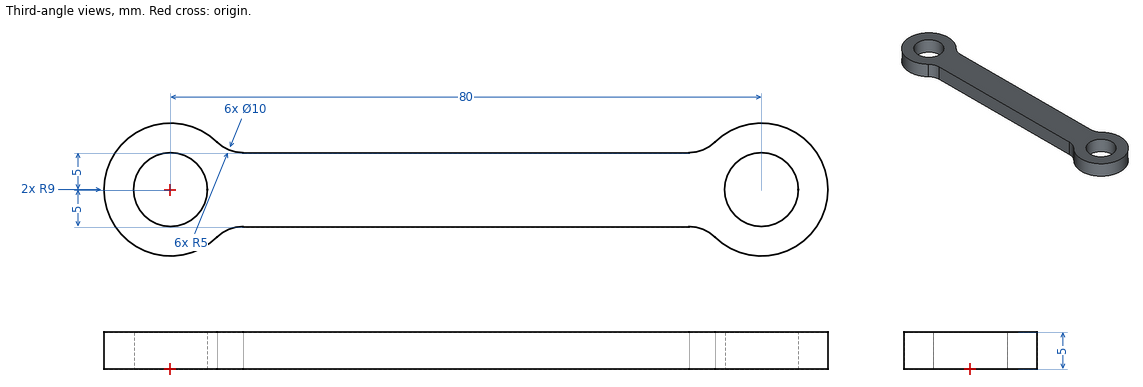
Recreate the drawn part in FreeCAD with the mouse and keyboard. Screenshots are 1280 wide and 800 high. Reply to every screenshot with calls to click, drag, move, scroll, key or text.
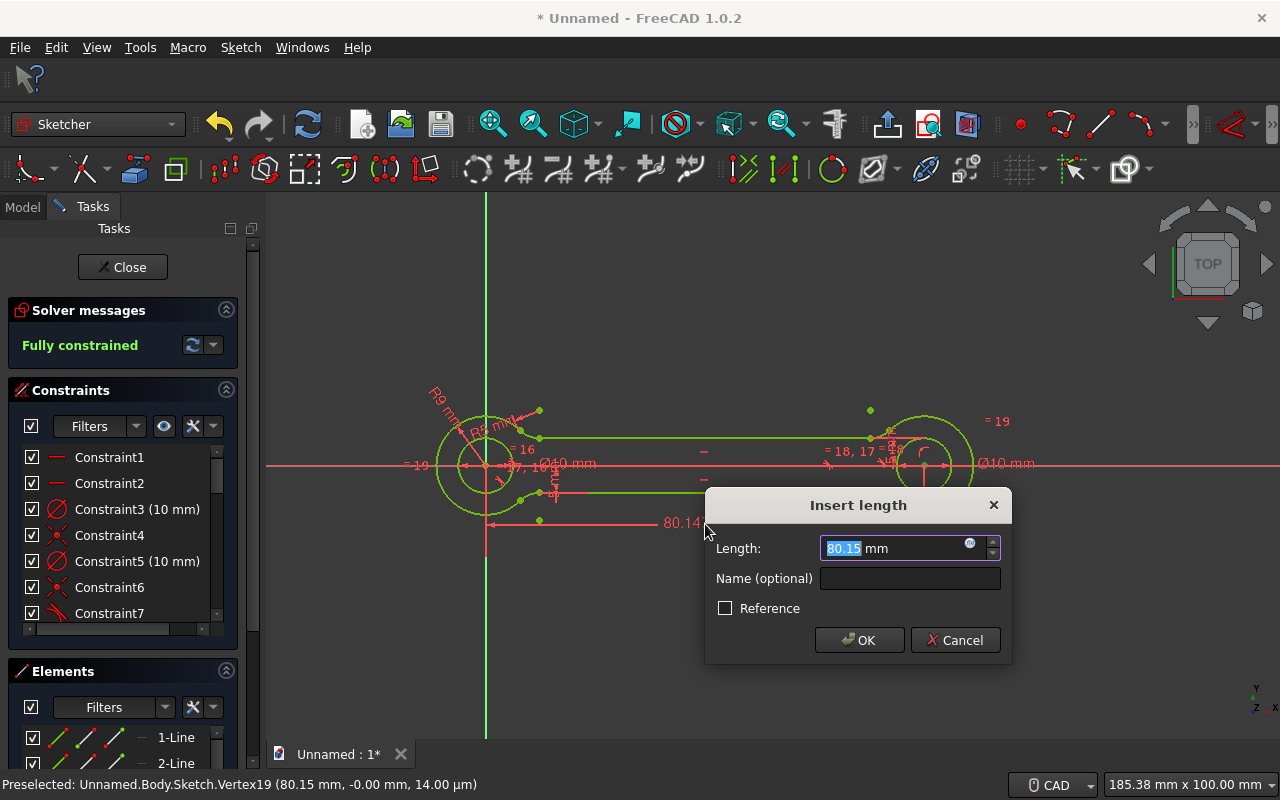
text(80)
key(Return)
key(Escape)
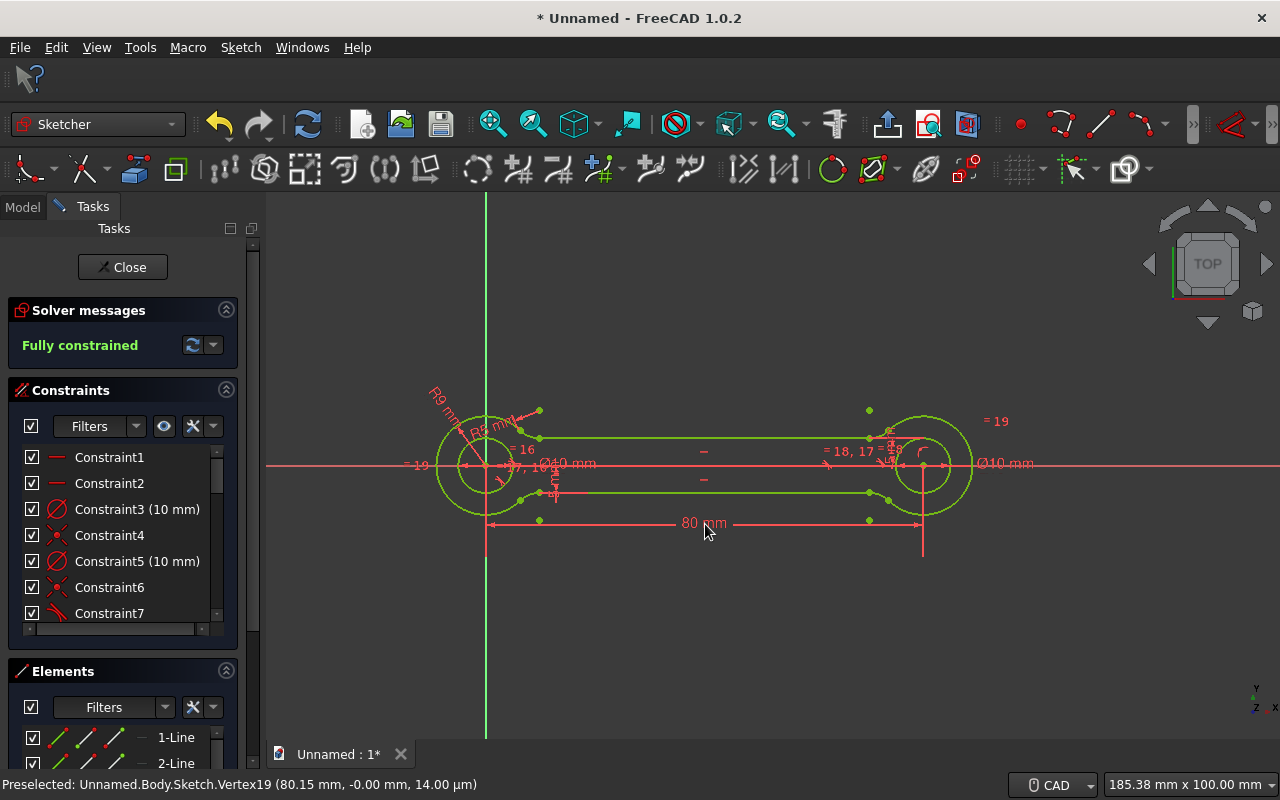
click(123, 267)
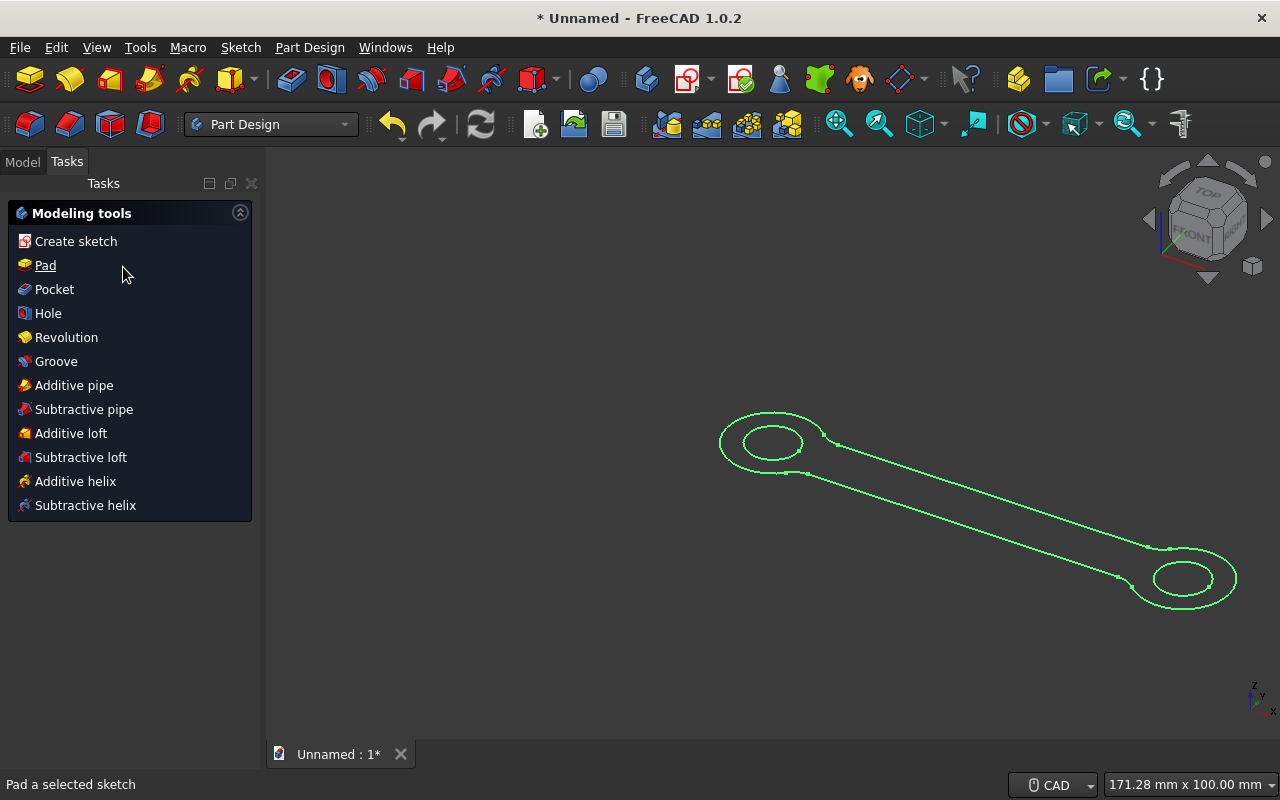
click(30, 80)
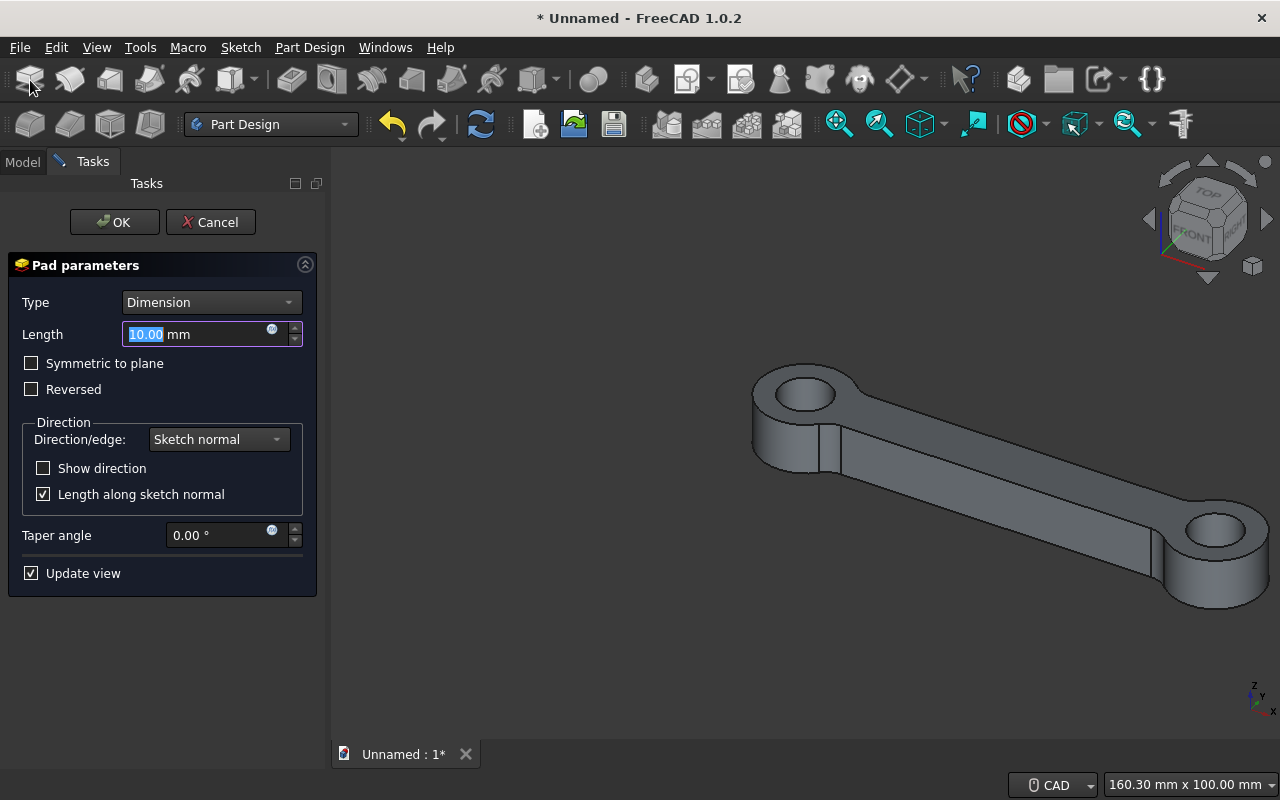
text(5)
key(Tab)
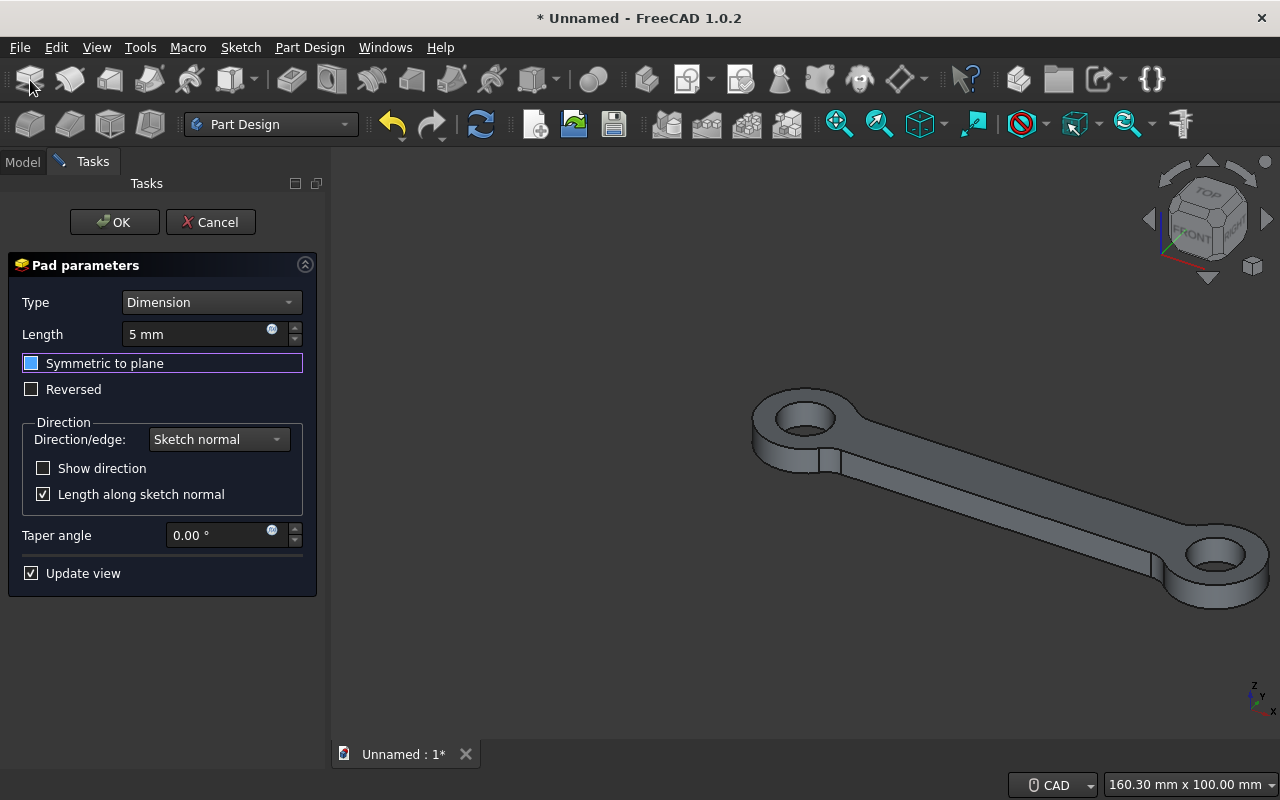
click(115, 222)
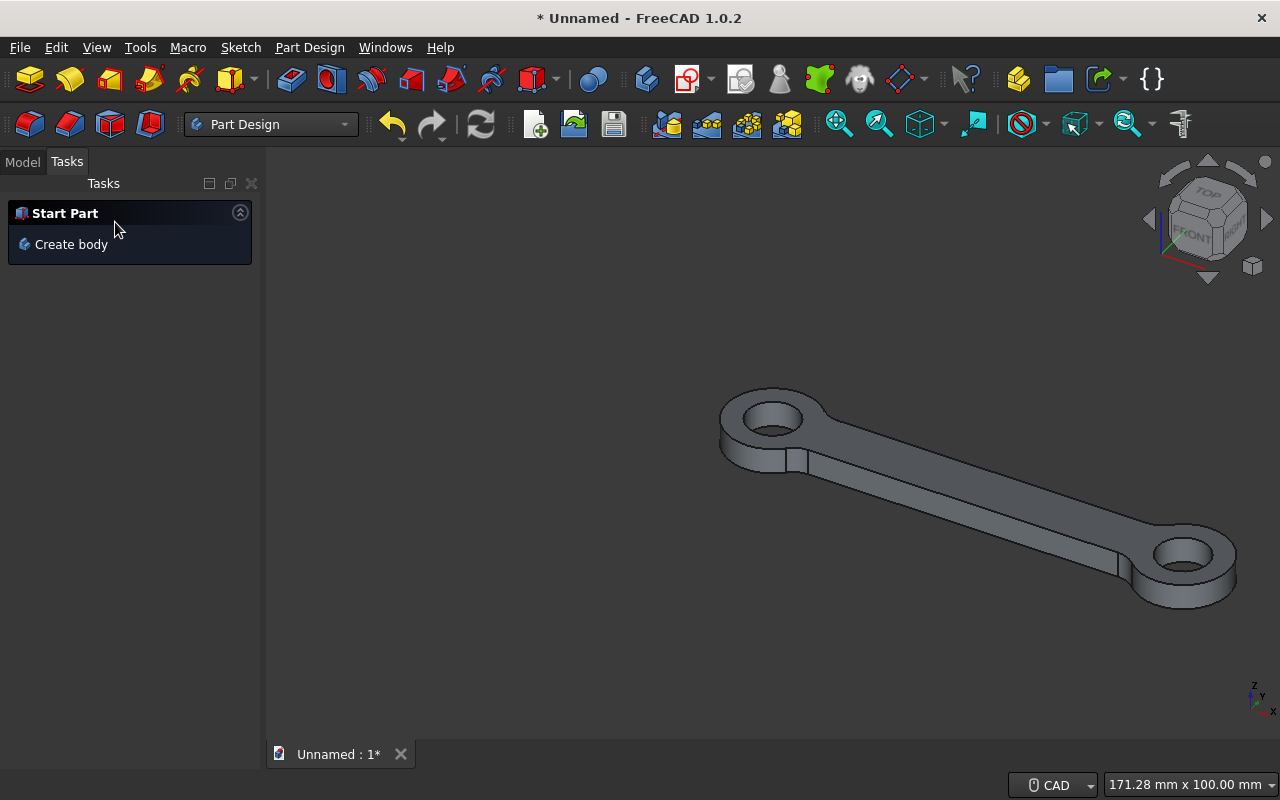
key(0)